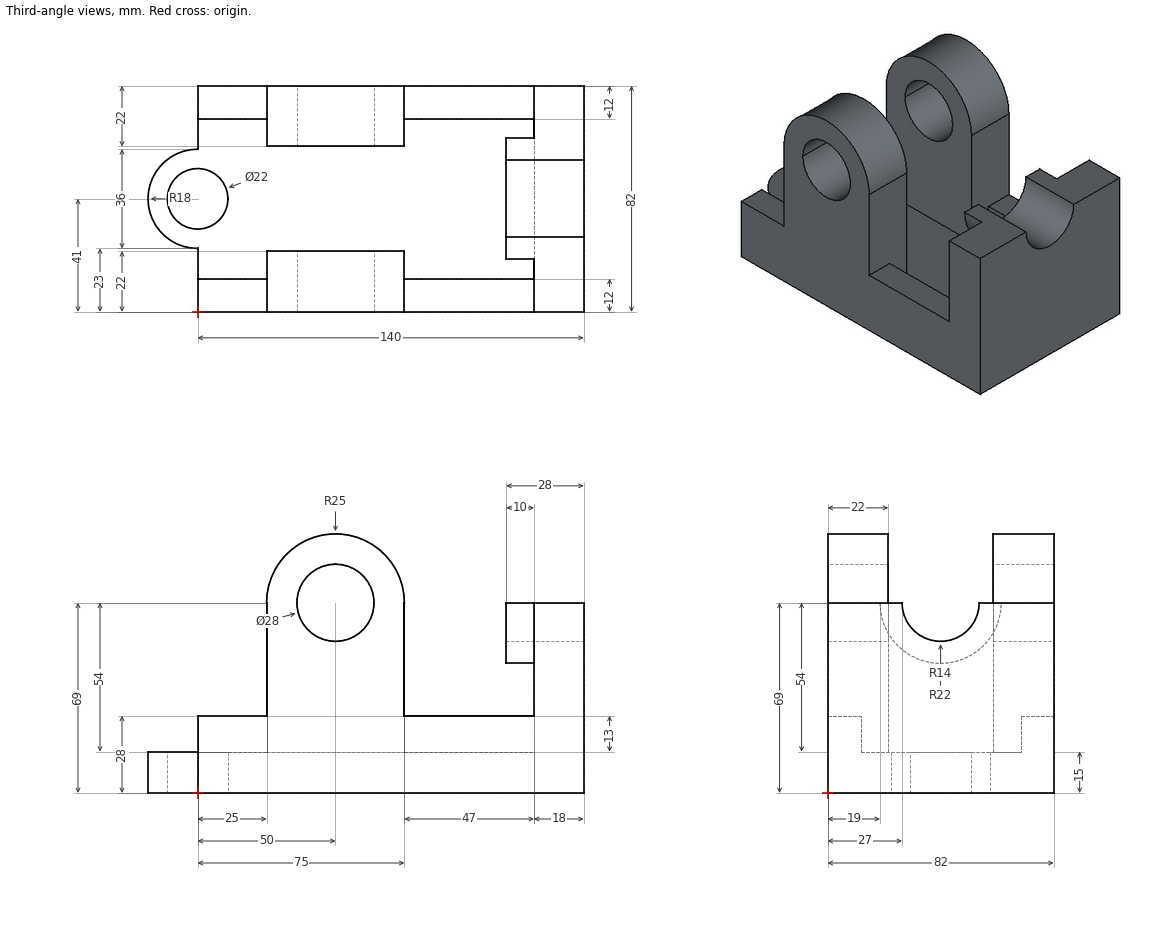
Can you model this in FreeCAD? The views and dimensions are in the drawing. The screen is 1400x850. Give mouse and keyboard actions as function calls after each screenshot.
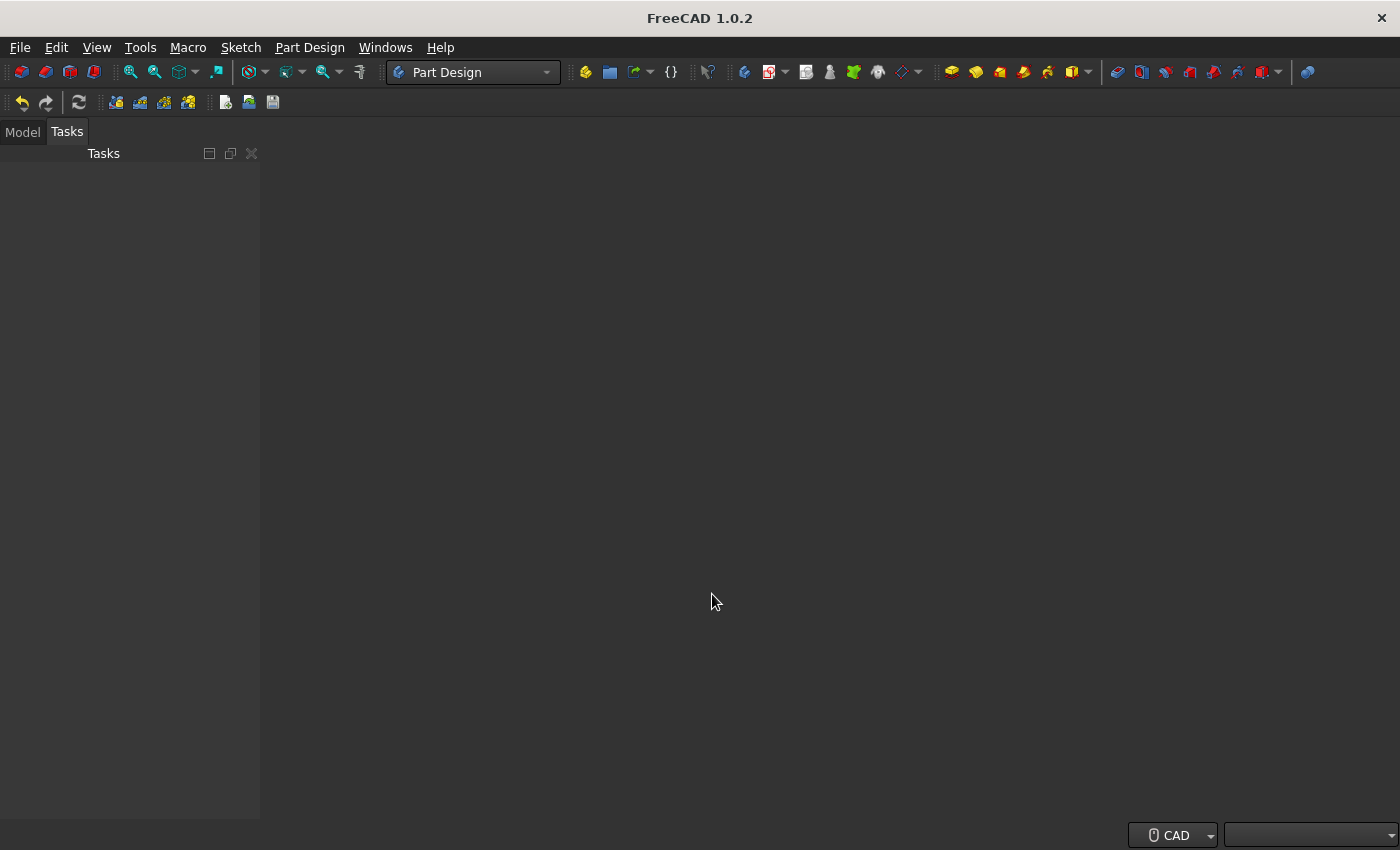
click(226, 102)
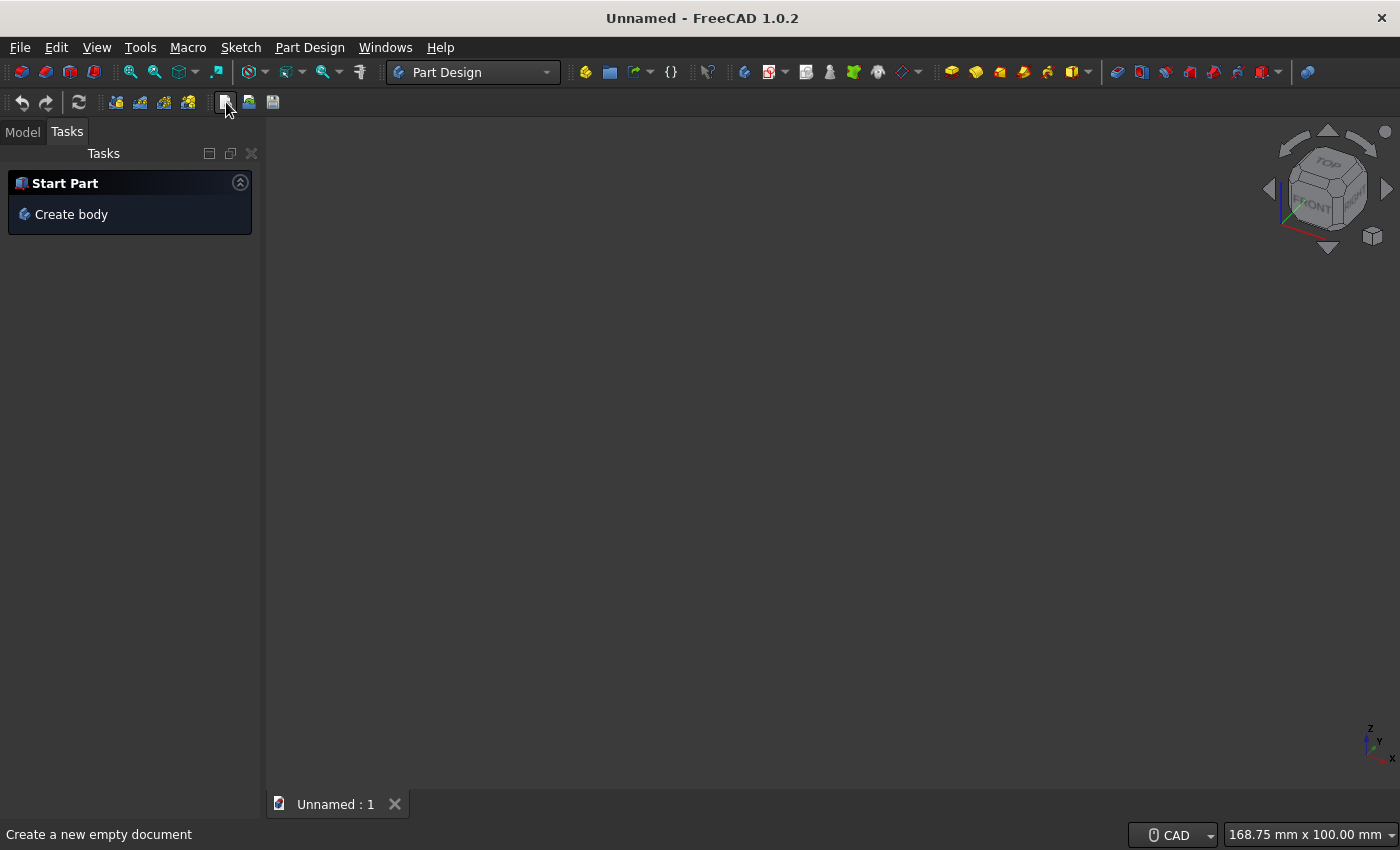
click(770, 72)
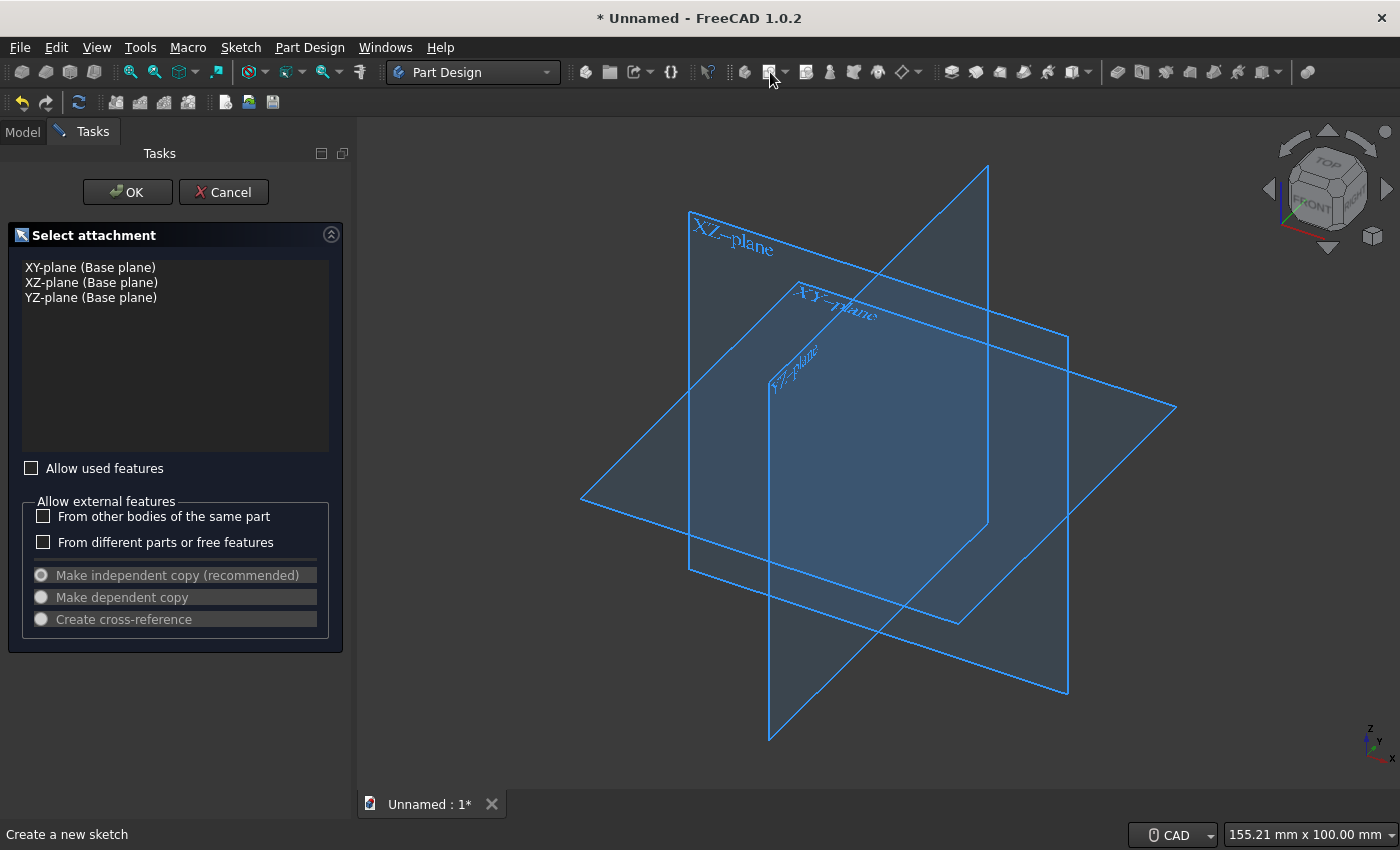
click(82, 268)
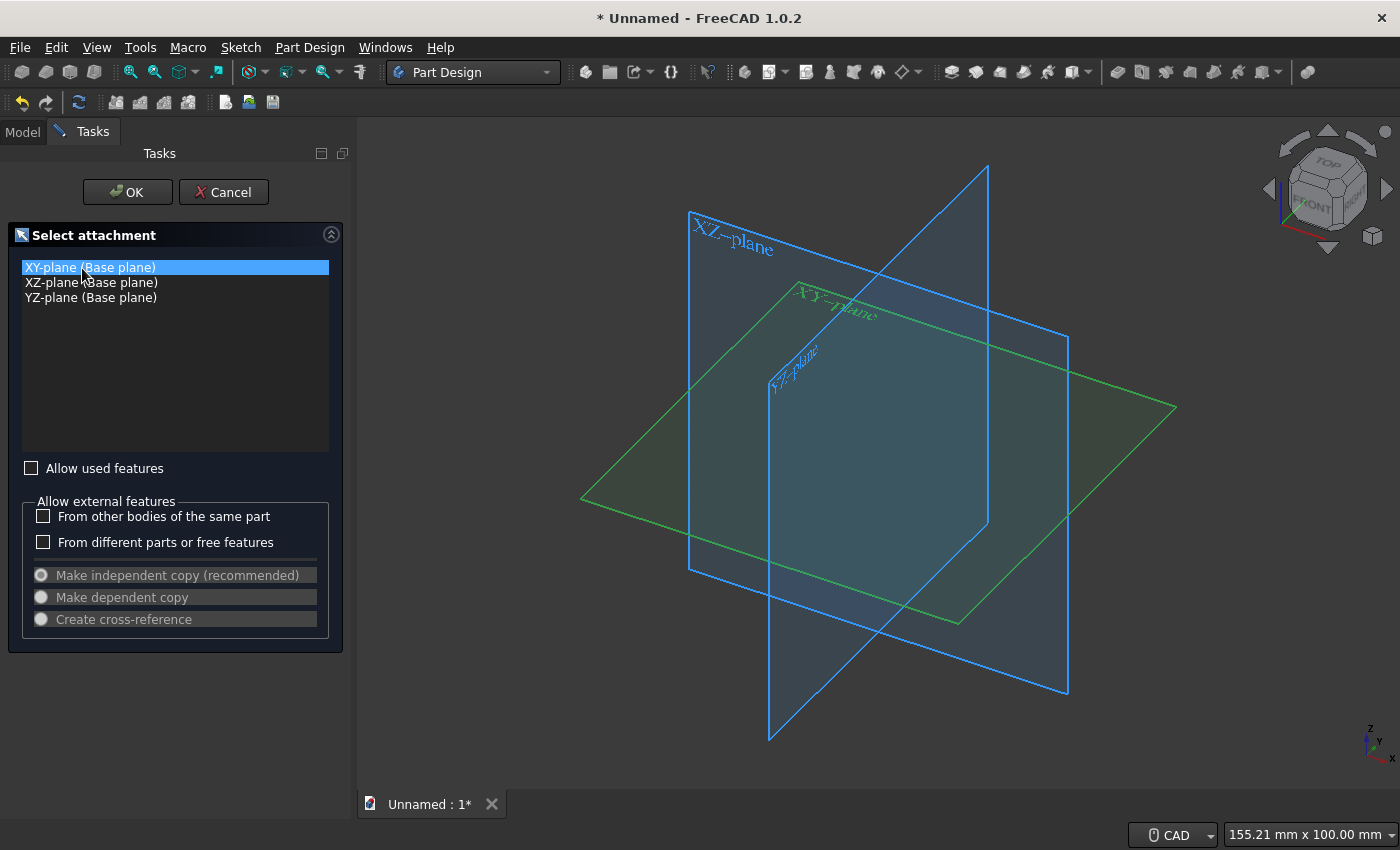
click(128, 192)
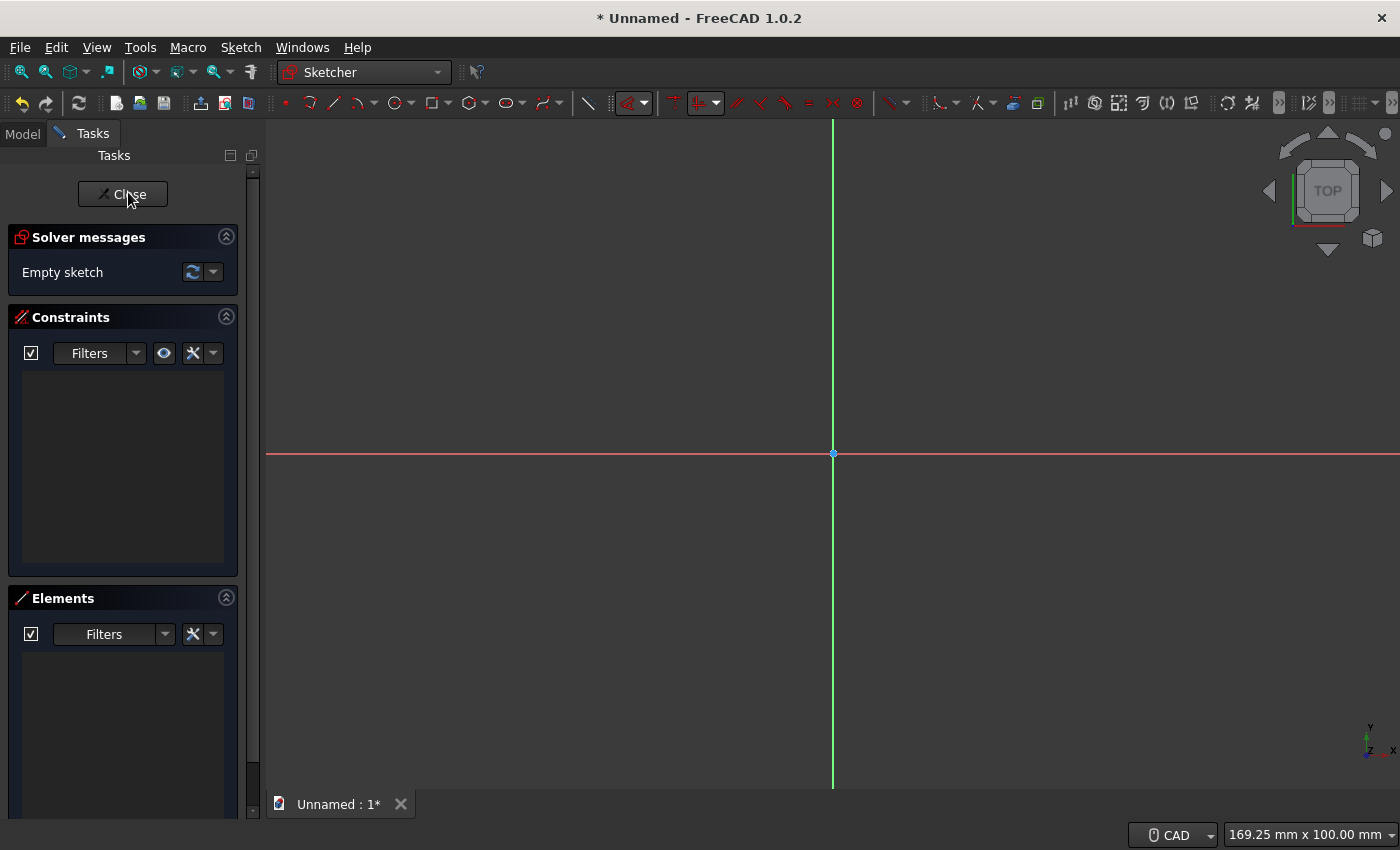
scroll(294, 761, down, 3)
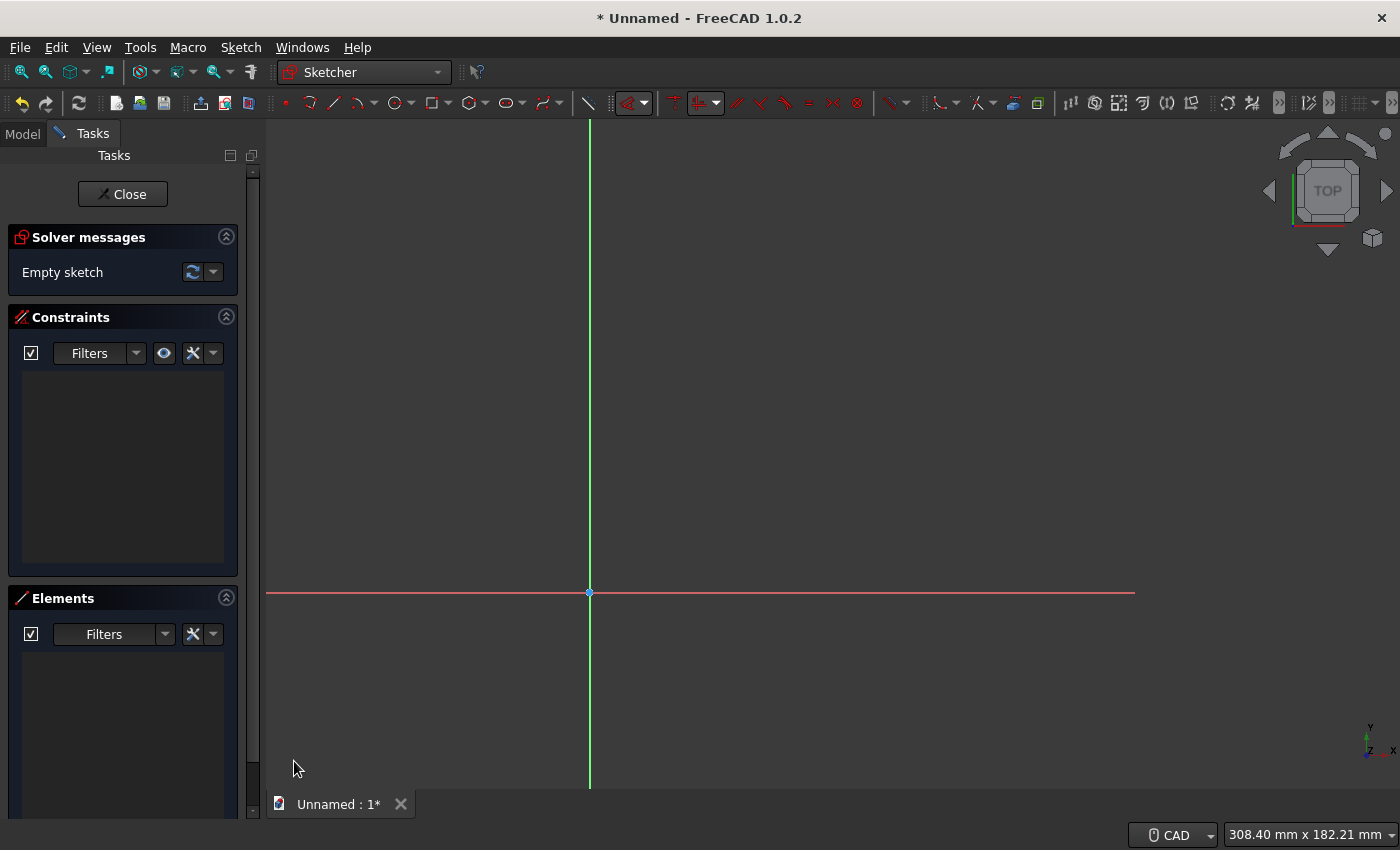
click(432, 104)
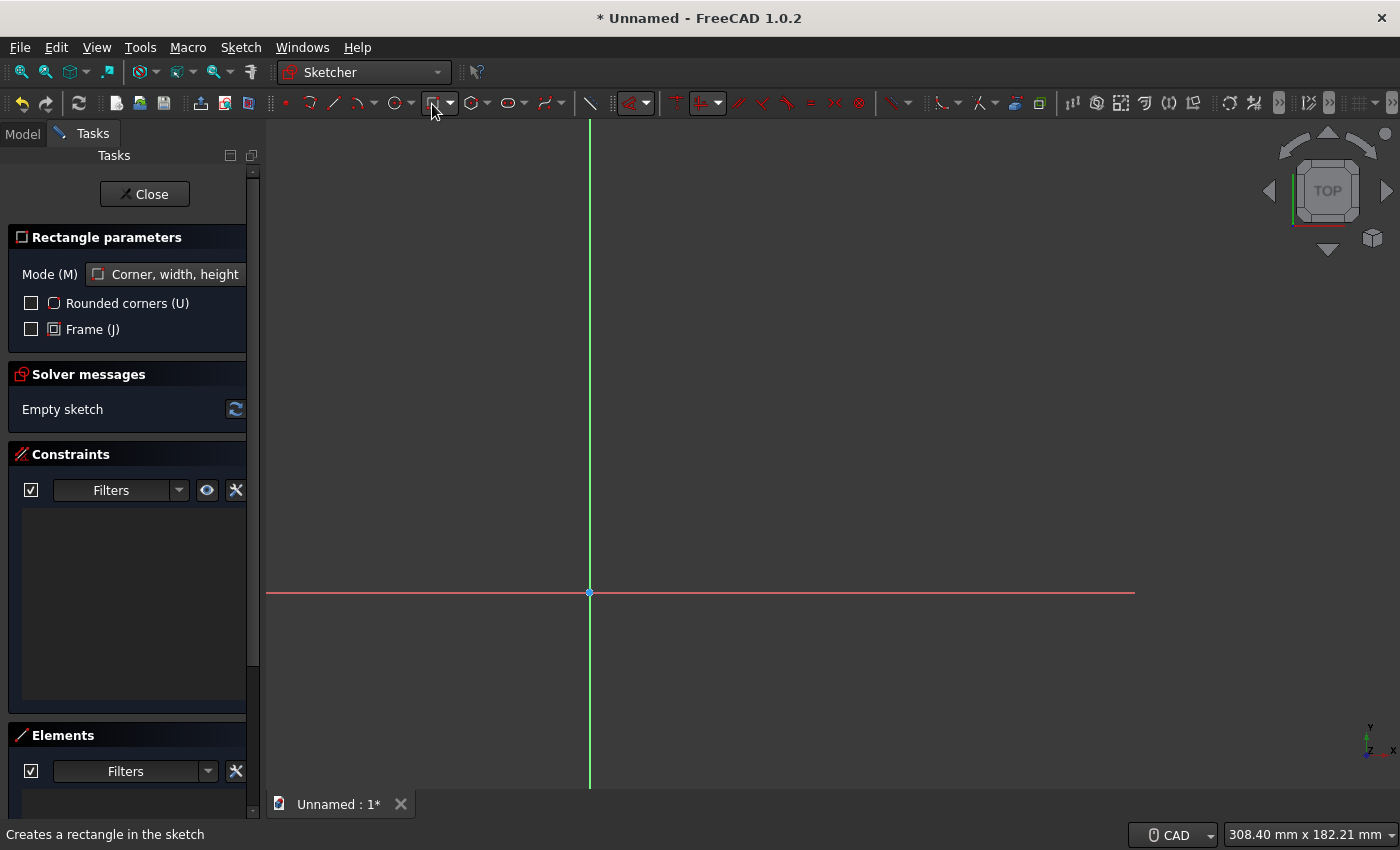
click(590, 593)
click(1105, 291)
key(Escape)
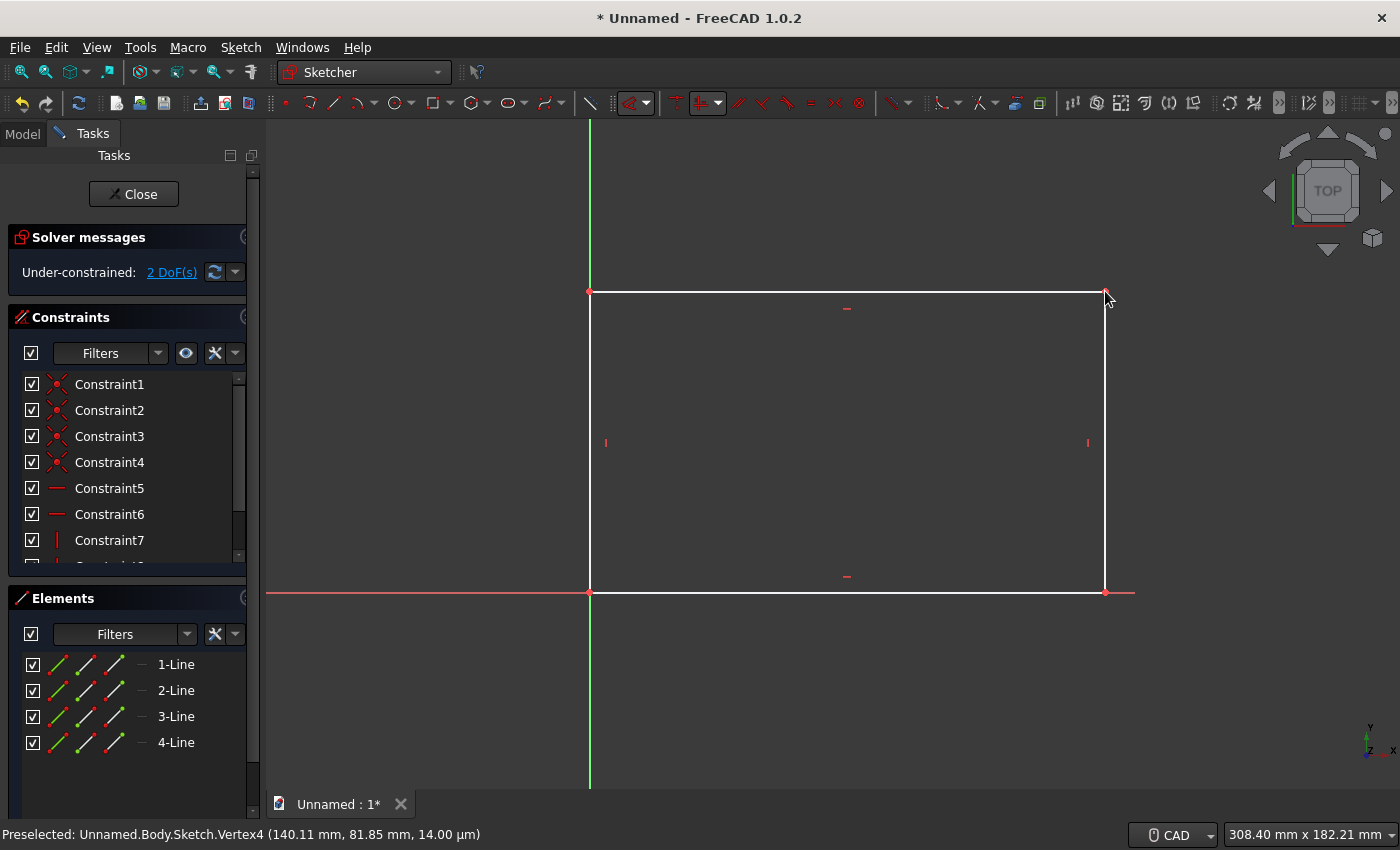
click(630, 104)